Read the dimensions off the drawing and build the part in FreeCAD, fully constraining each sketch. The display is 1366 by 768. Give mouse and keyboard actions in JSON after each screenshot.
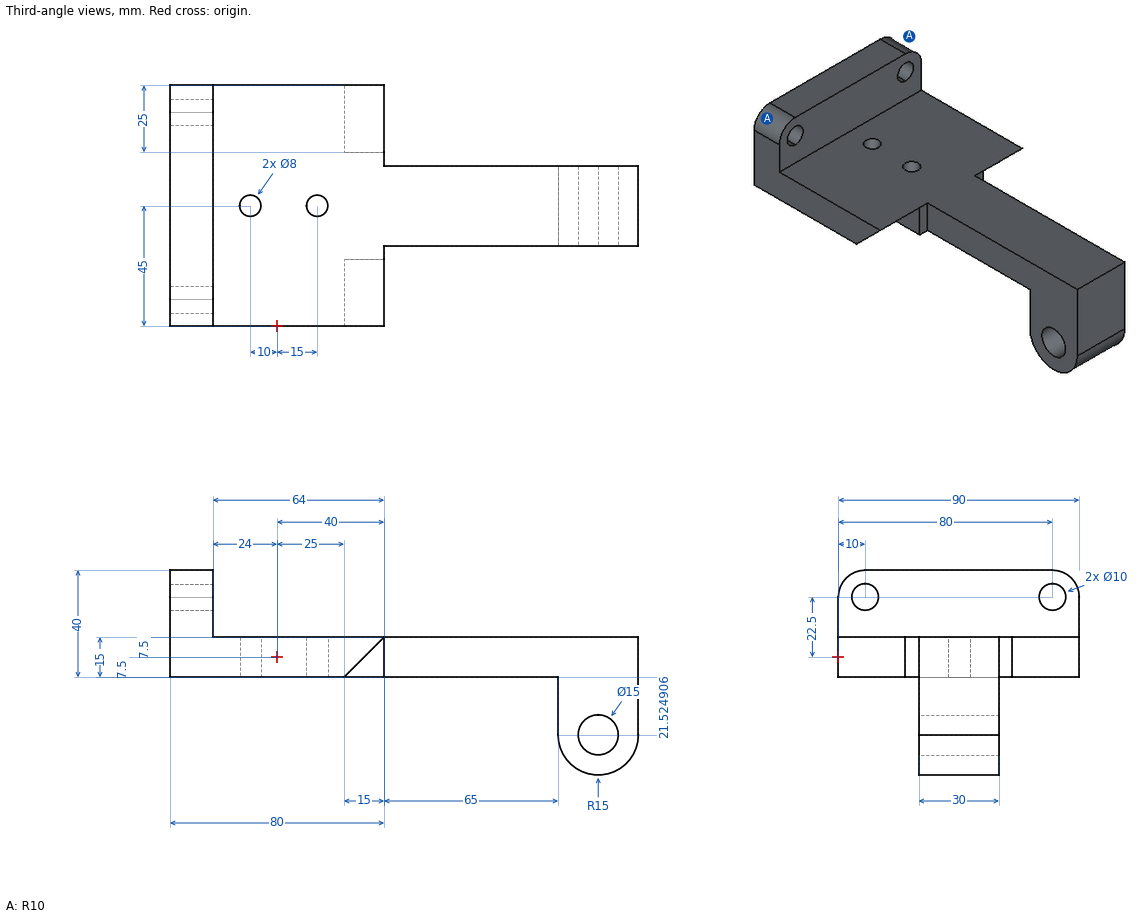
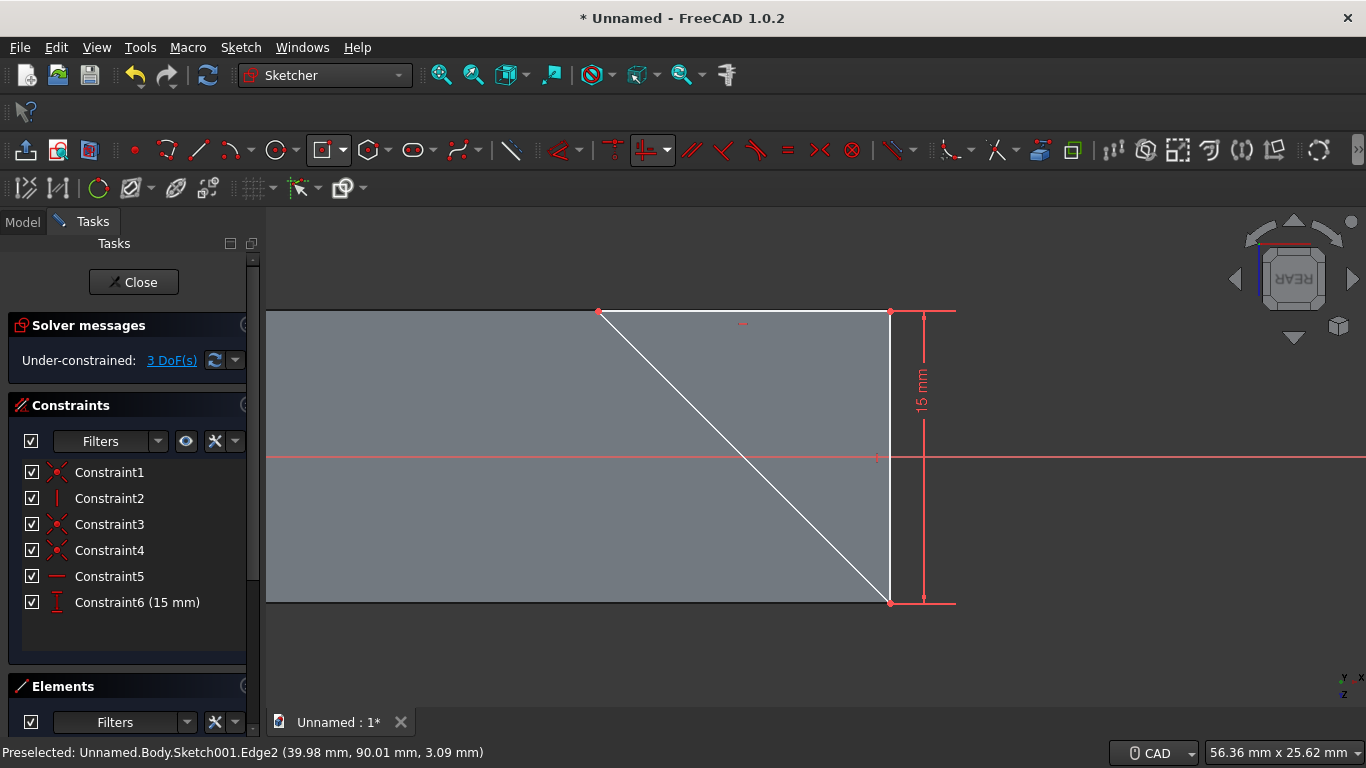
{"action": "left_click", "coordinate": [802, 311]}
{"action": "left_click", "coordinate": [744, 277]}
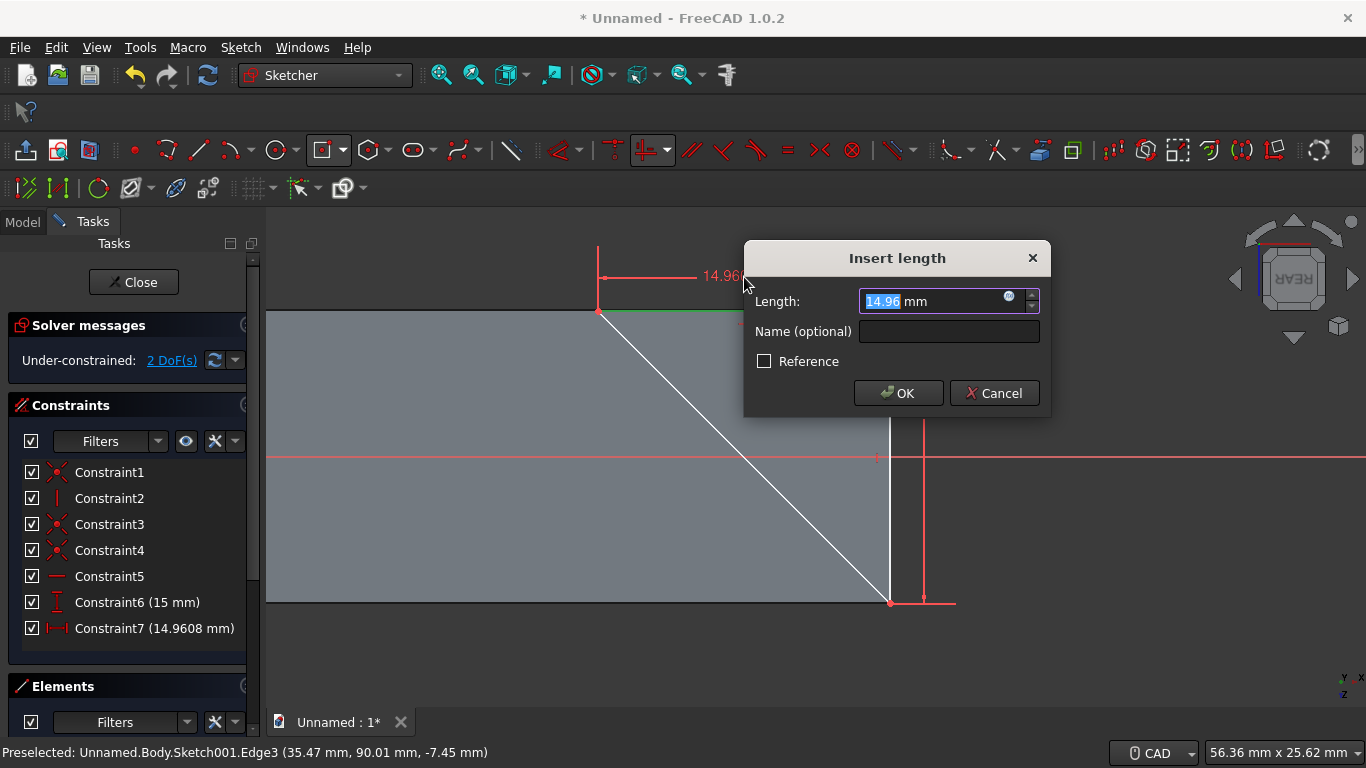
{"action": "type", "text": "15"}
{"action": "key", "text": "Return"}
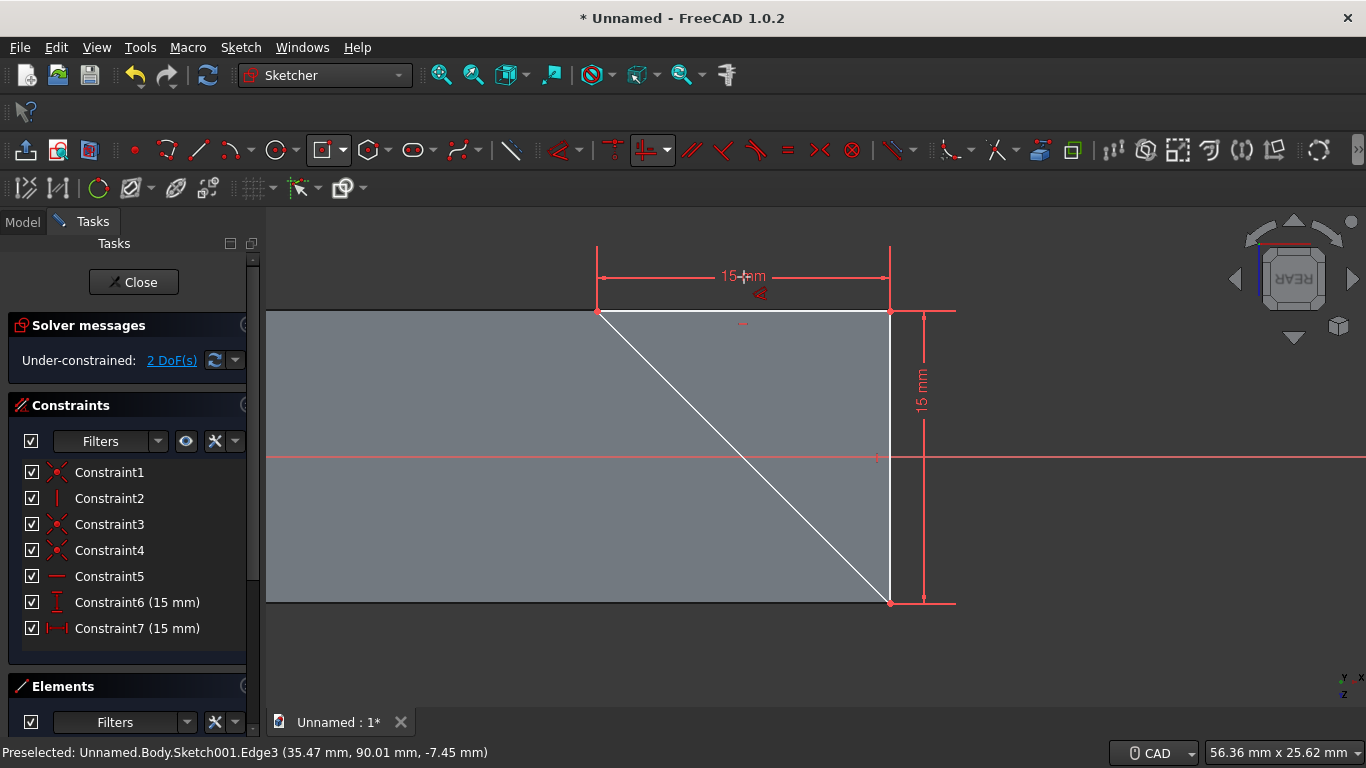
{"action": "left_click", "coordinate": [597, 311]}
{"action": "left_click", "coordinate": [446, 277]}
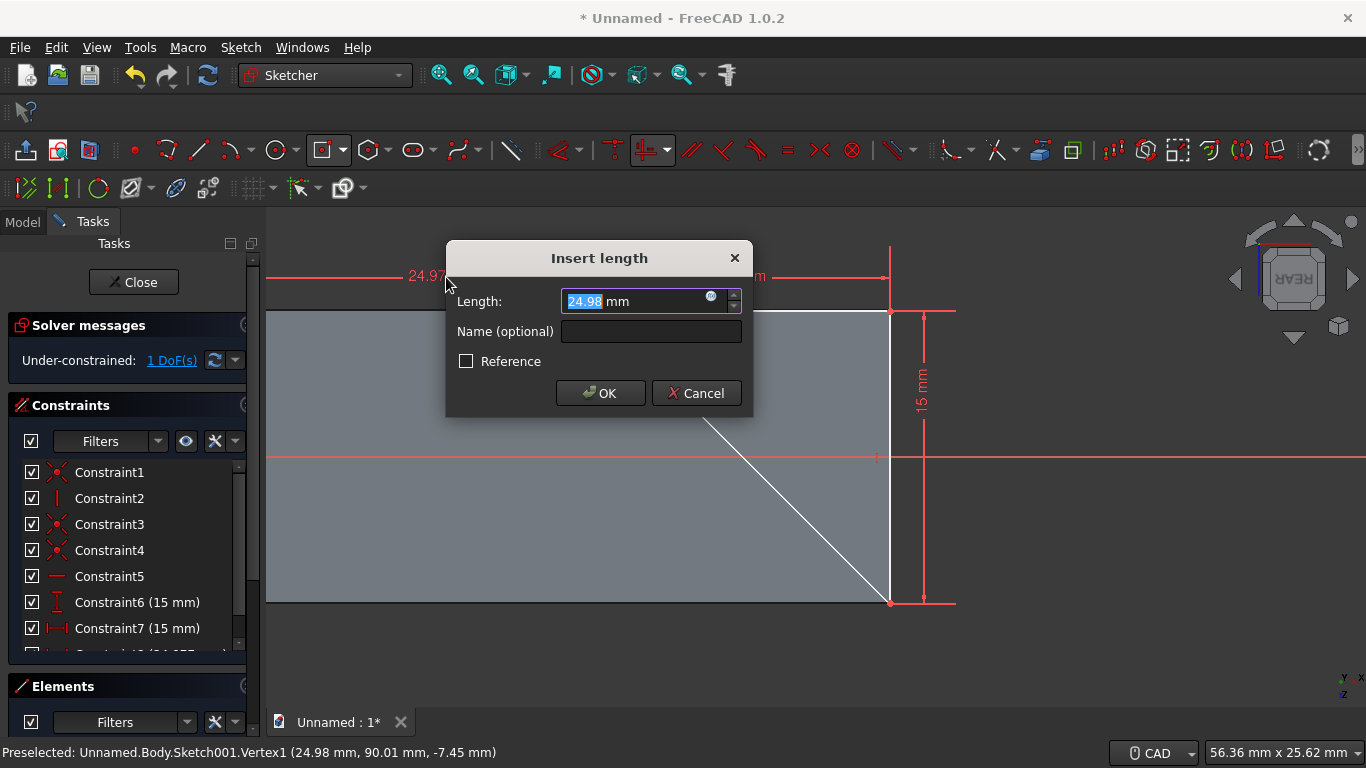
{"action": "type", "text": "25"}
{"action": "key", "text": "Return"}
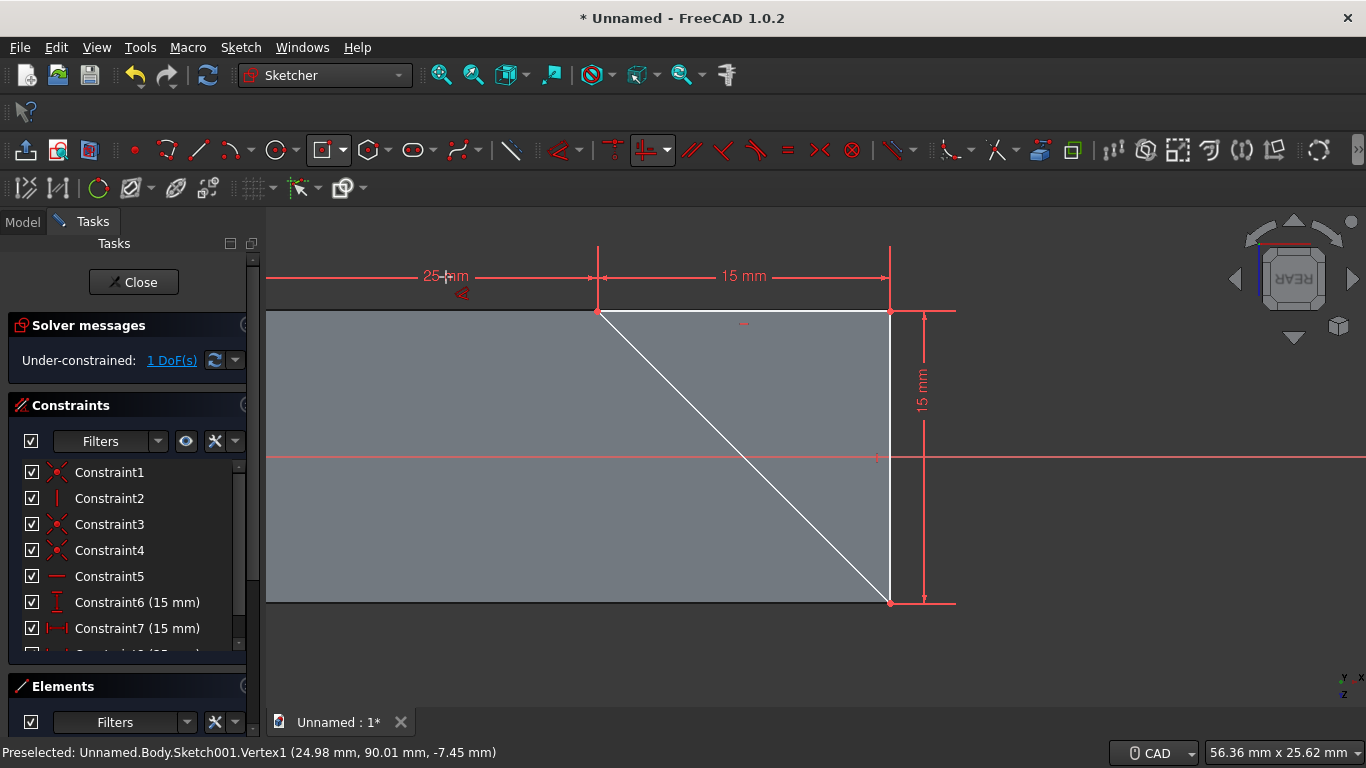
{"action": "left_click", "coordinate": [598, 311]}
{"action": "left_click", "coordinate": [632, 384]}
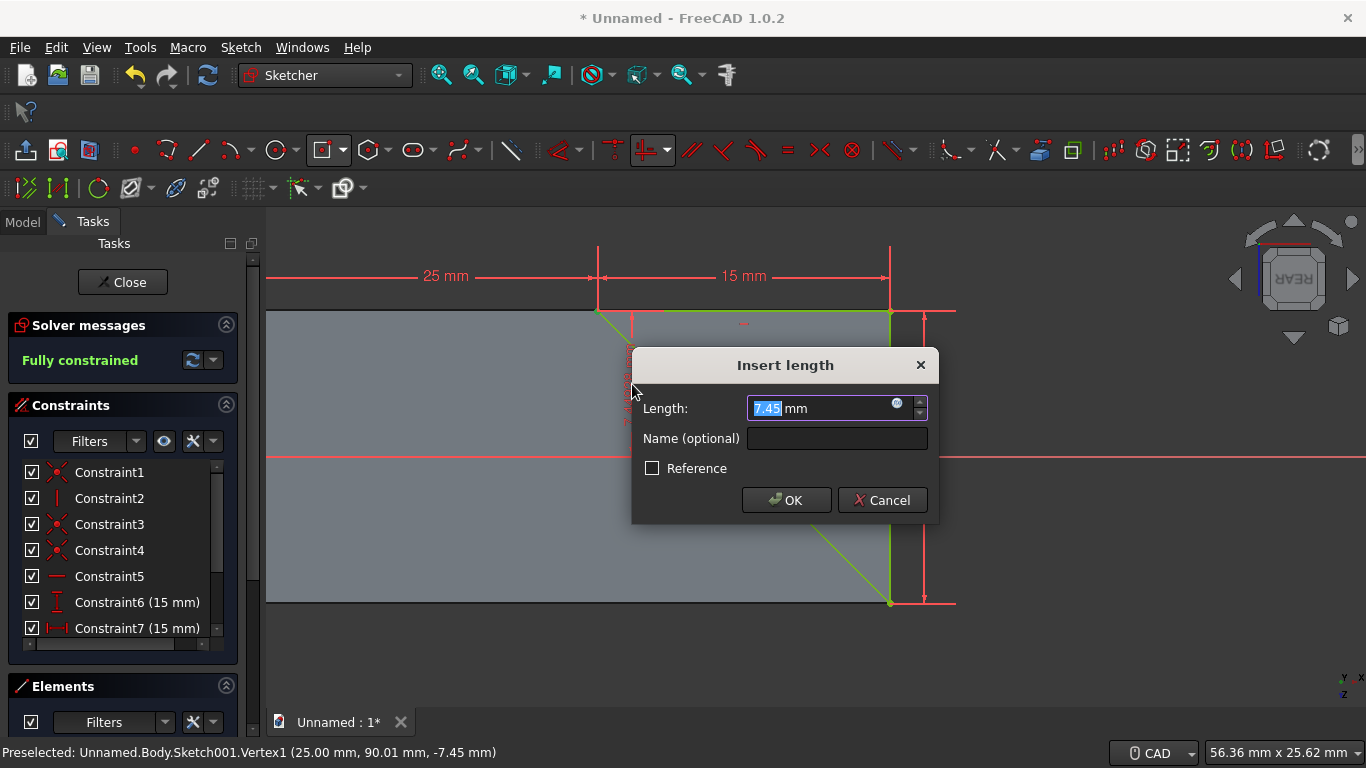
{"action": "type", "text": "7.5"}
{"action": "key", "text": "Return"}
{"action": "key", "text": "Escape"}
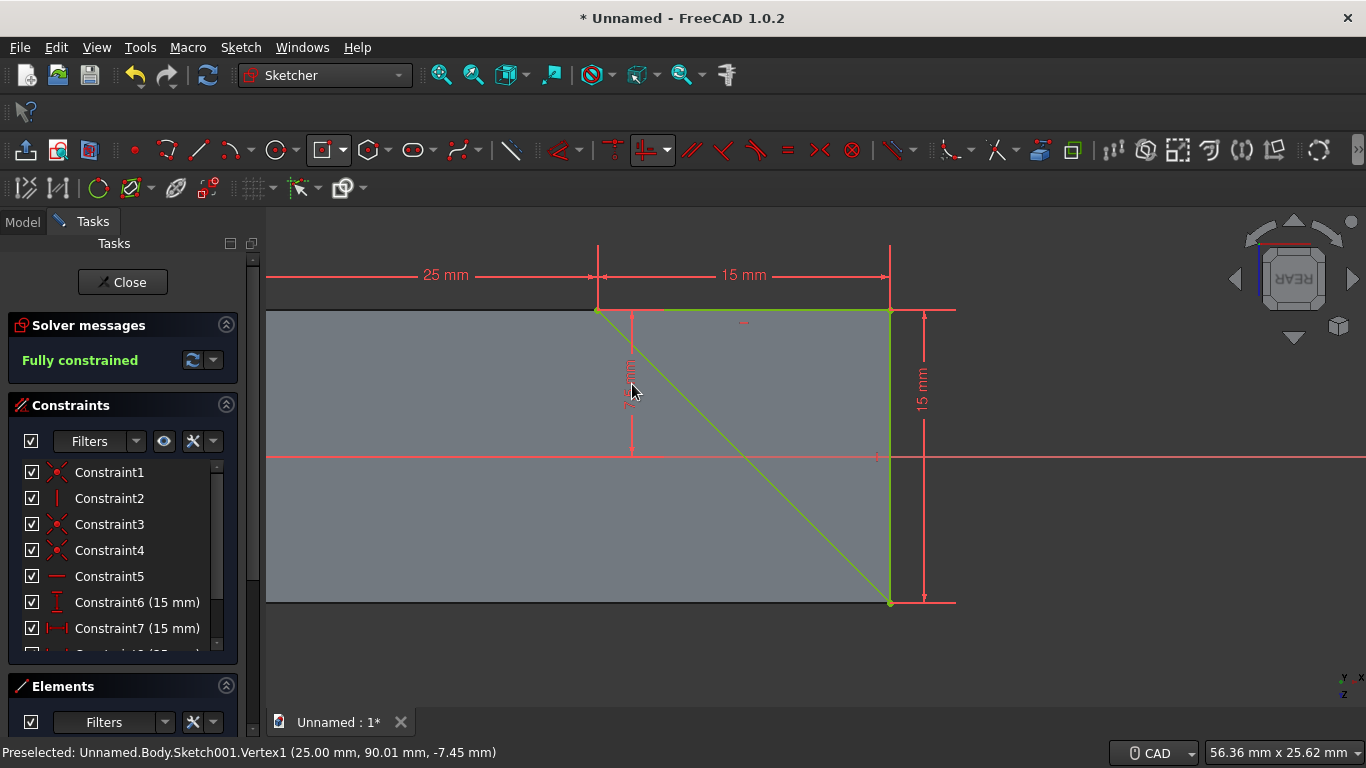
{"action": "left_click", "coordinate": [123, 282]}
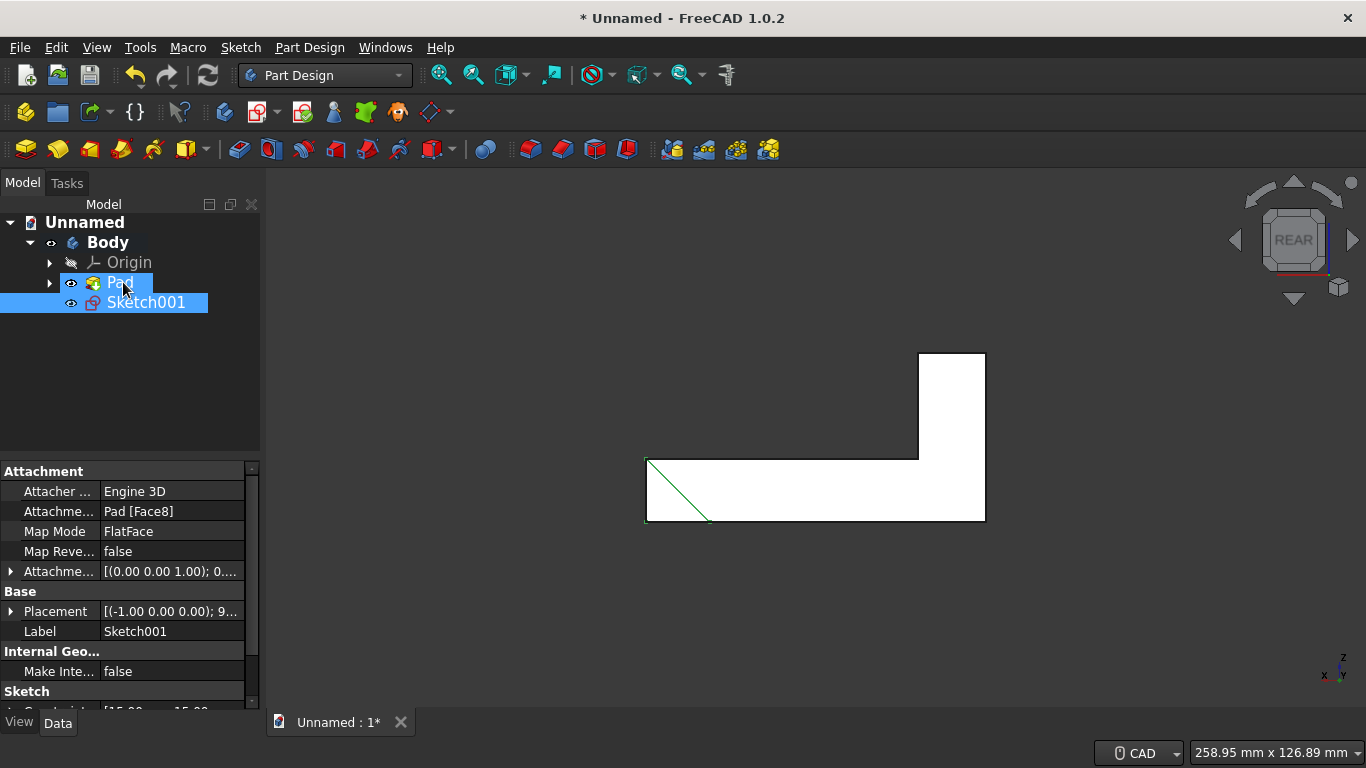
{"action": "left_click", "coordinate": [240, 150]}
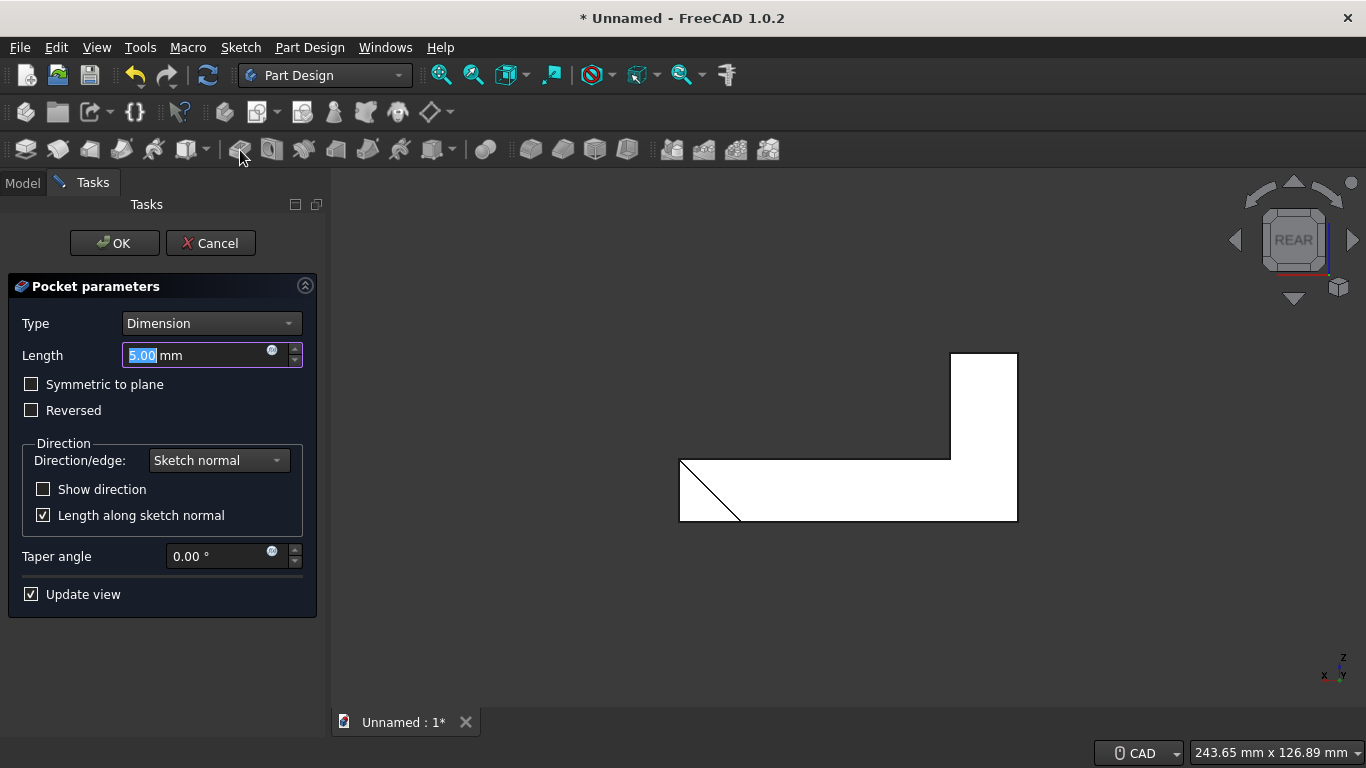
{"action": "type", "text": "25"}
{"action": "key", "text": "Tab"}